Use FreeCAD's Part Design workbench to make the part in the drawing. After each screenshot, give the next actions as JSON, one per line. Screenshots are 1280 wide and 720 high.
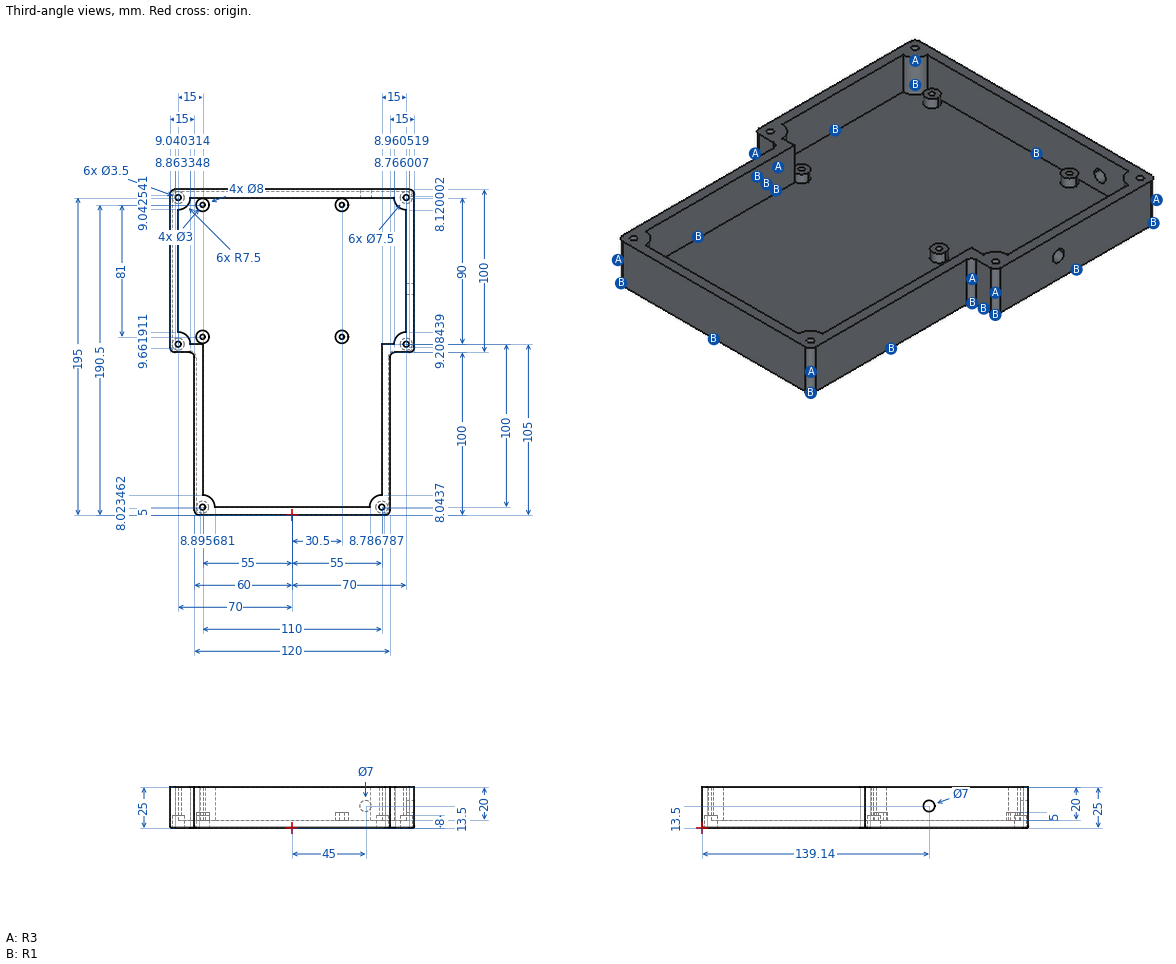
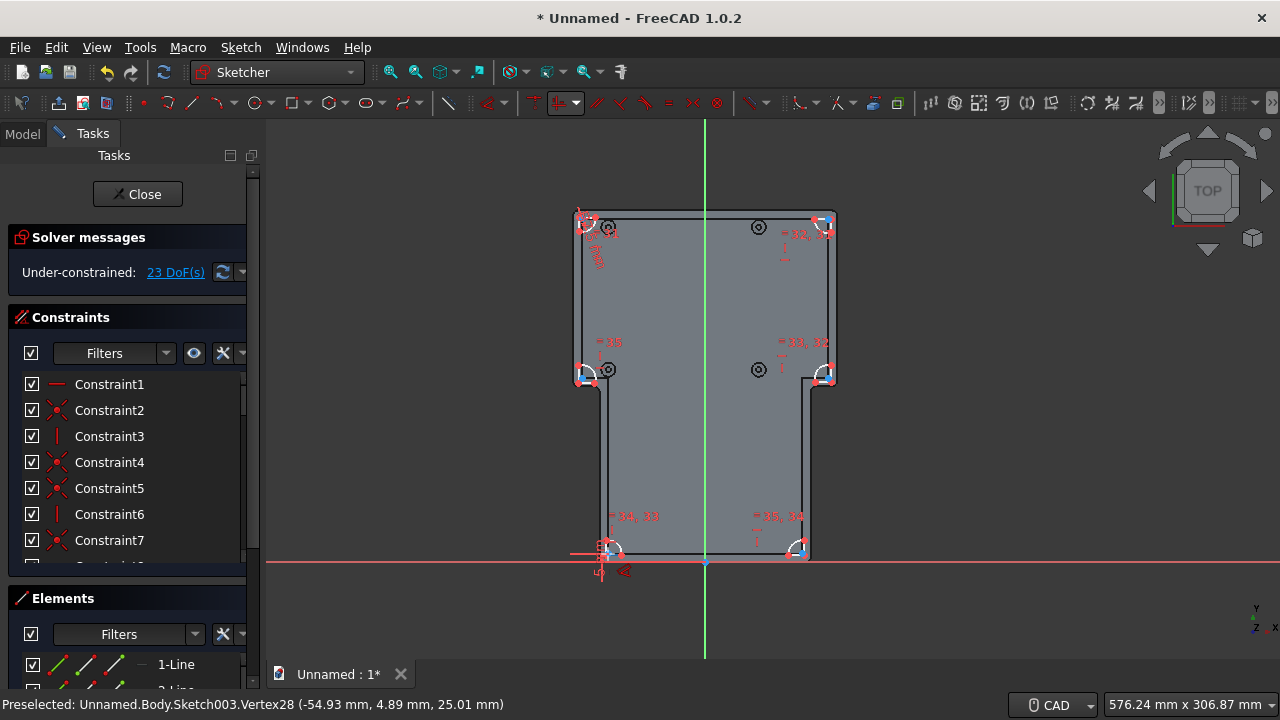
{"action": "scroll", "coordinate": [802, 554], "scroll_direction": "up", "scroll_amount": 8}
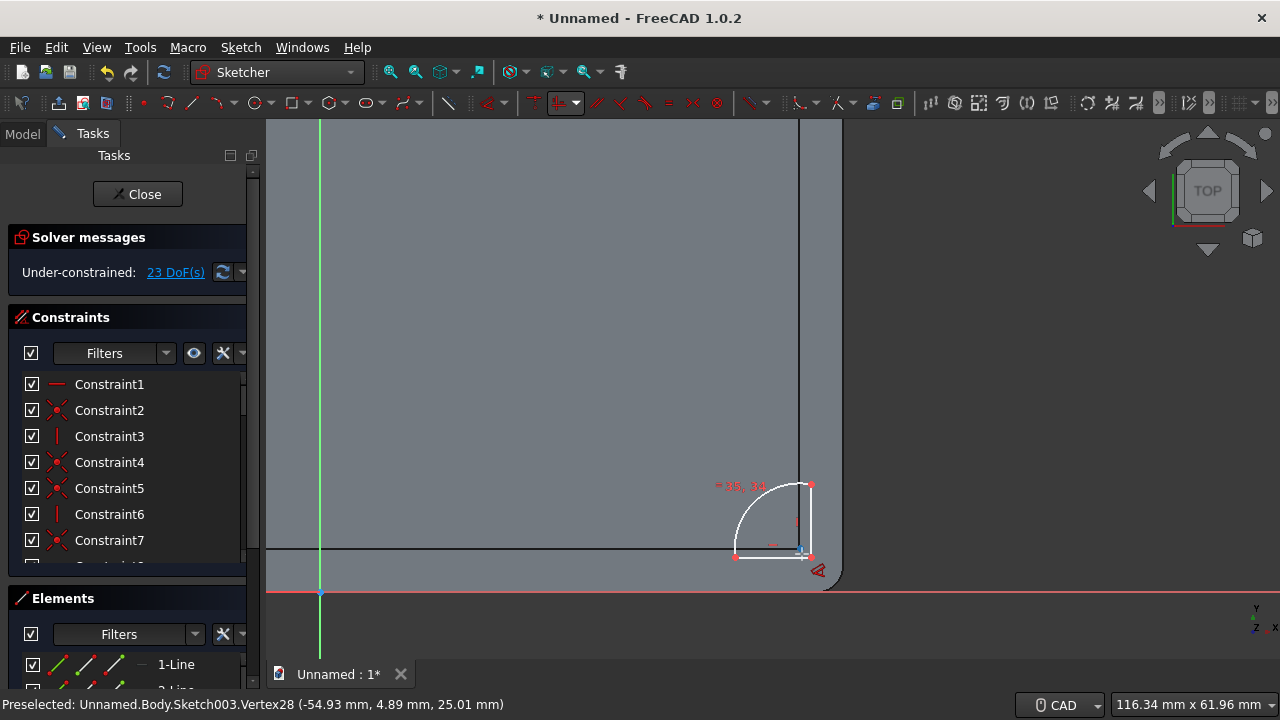
{"action": "left_click", "coordinate": [800, 549]}
{"action": "left_click", "coordinate": [834, 571]}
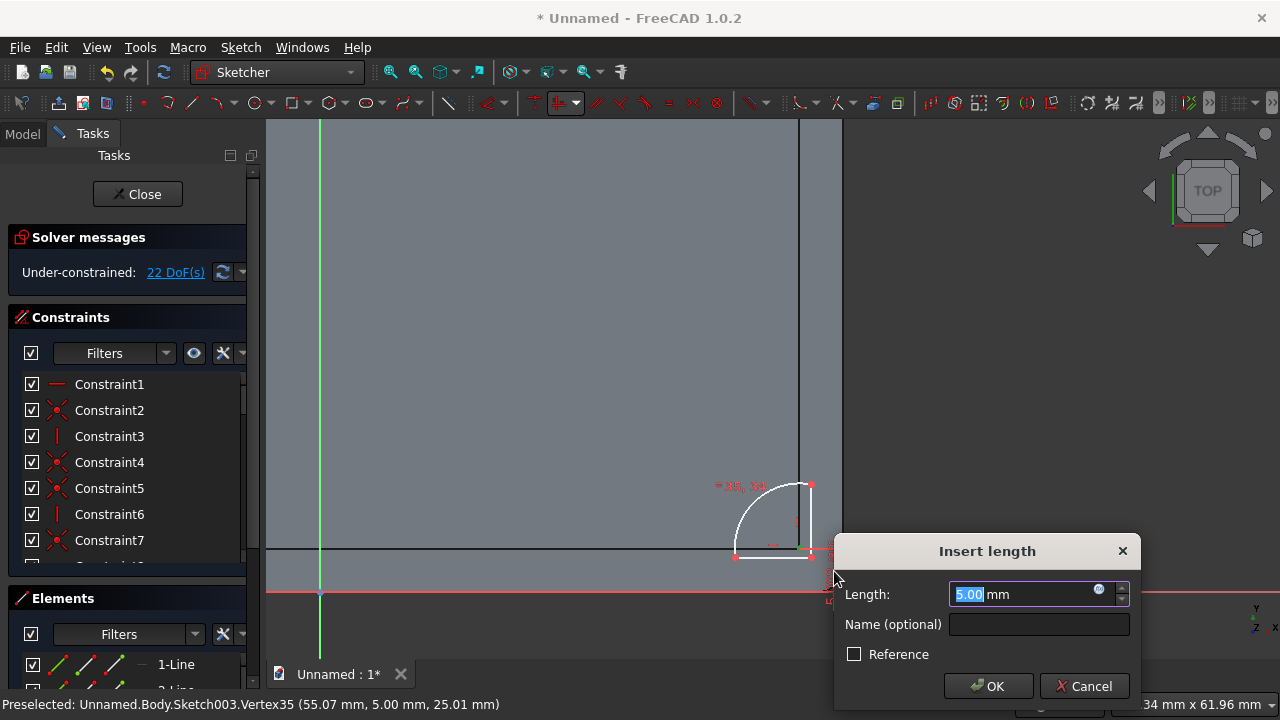
{"action": "type", "text": "5"}
{"action": "key", "text": "Return"}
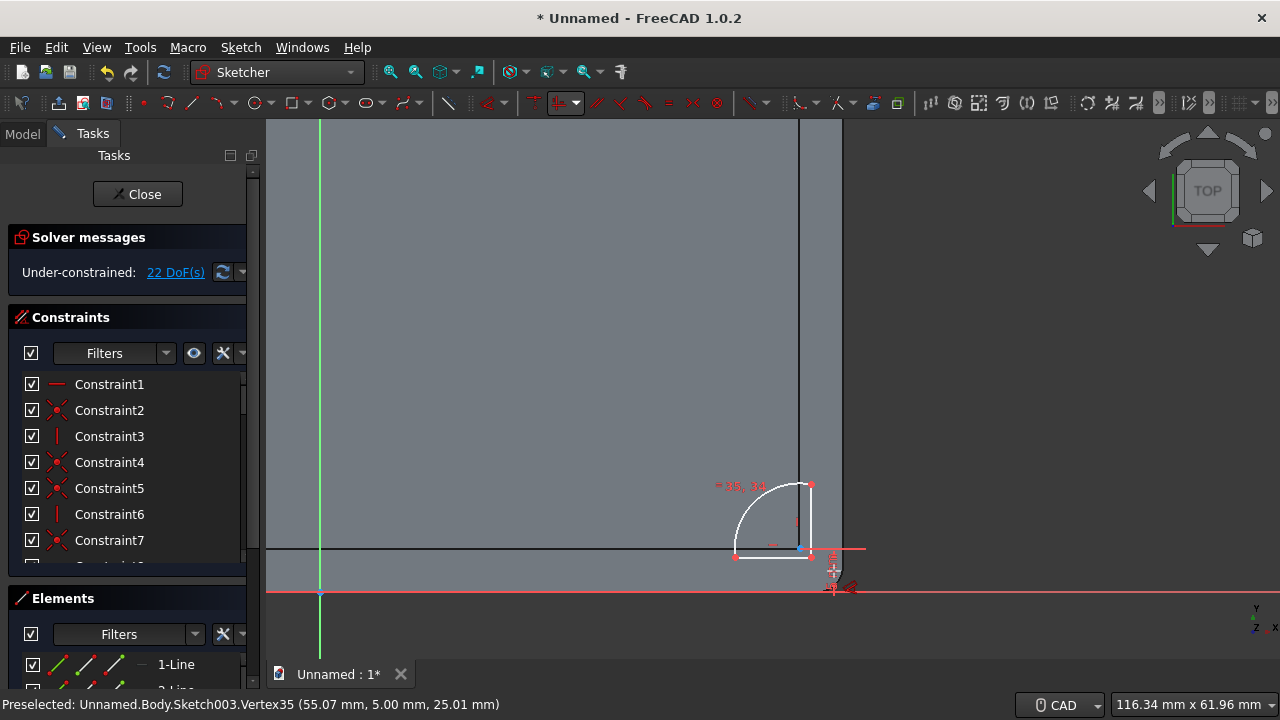
{"action": "scroll", "coordinate": [802, 554], "scroll_direction": "down", "scroll_amount": 8}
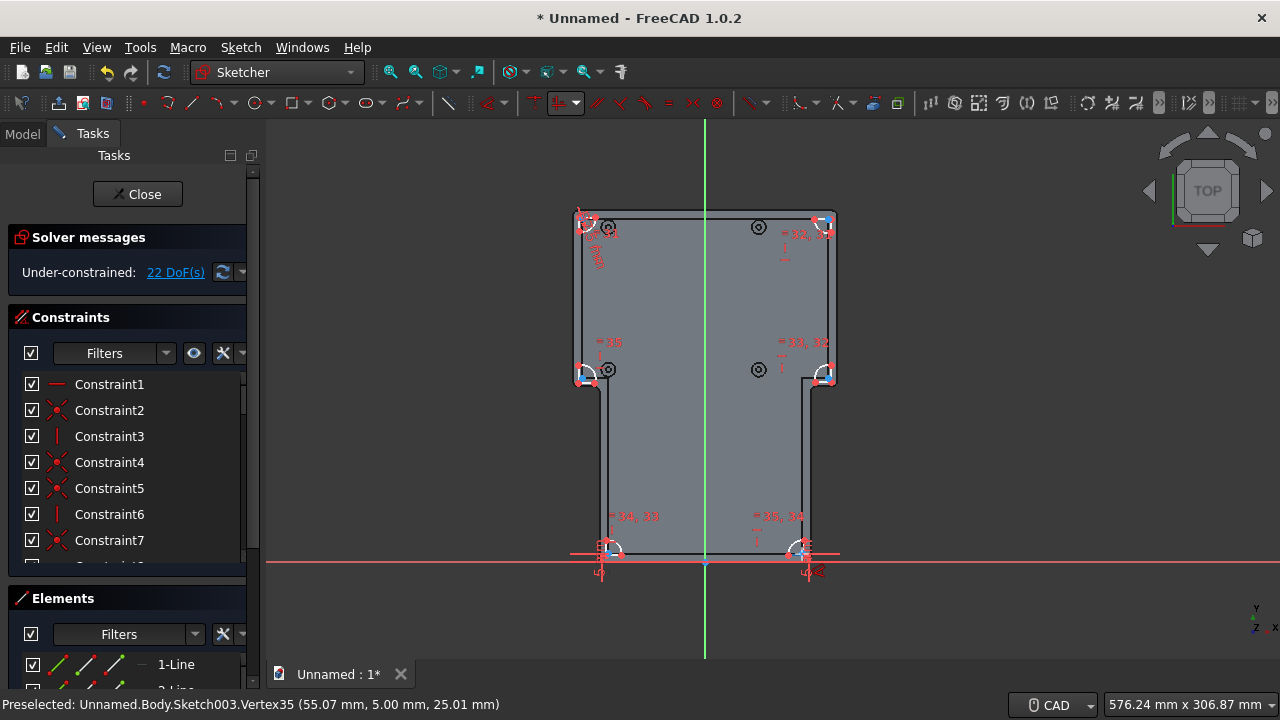
{"action": "scroll", "coordinate": [582, 219], "scroll_direction": "up", "scroll_amount": 7}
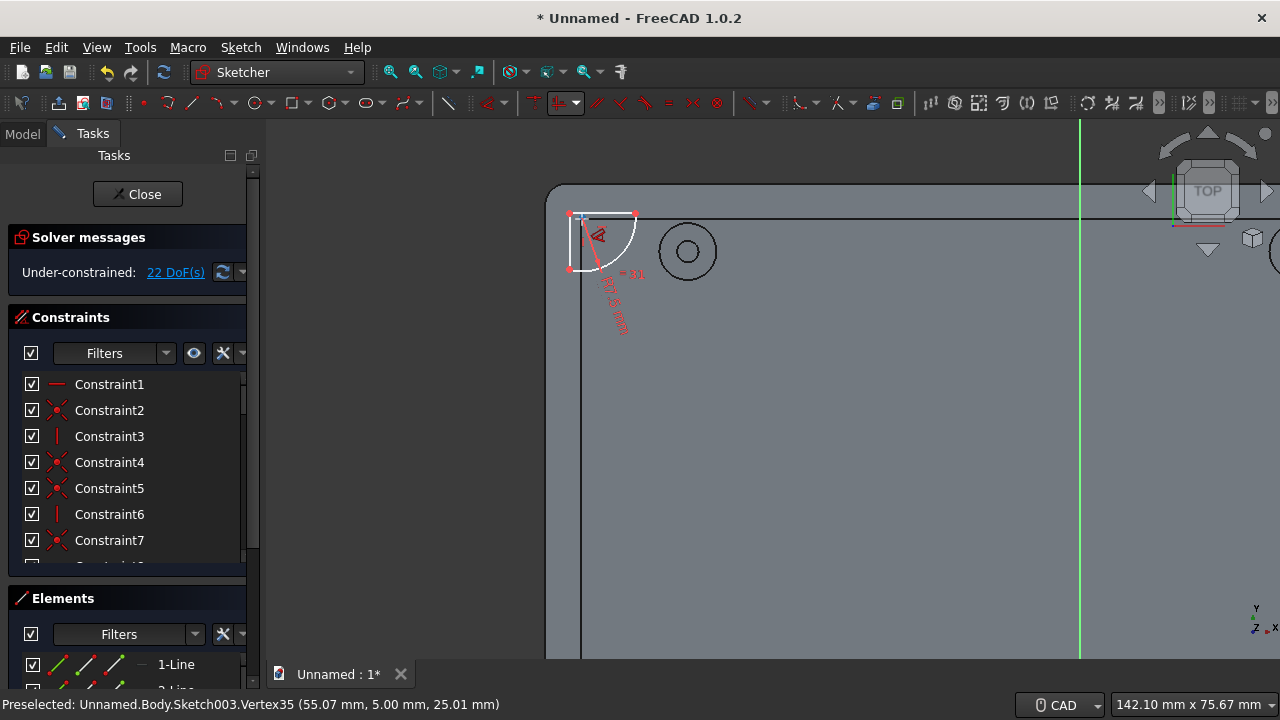
{"action": "left_click", "coordinate": [582, 218]}
{"action": "left_click", "coordinate": [831, 184]}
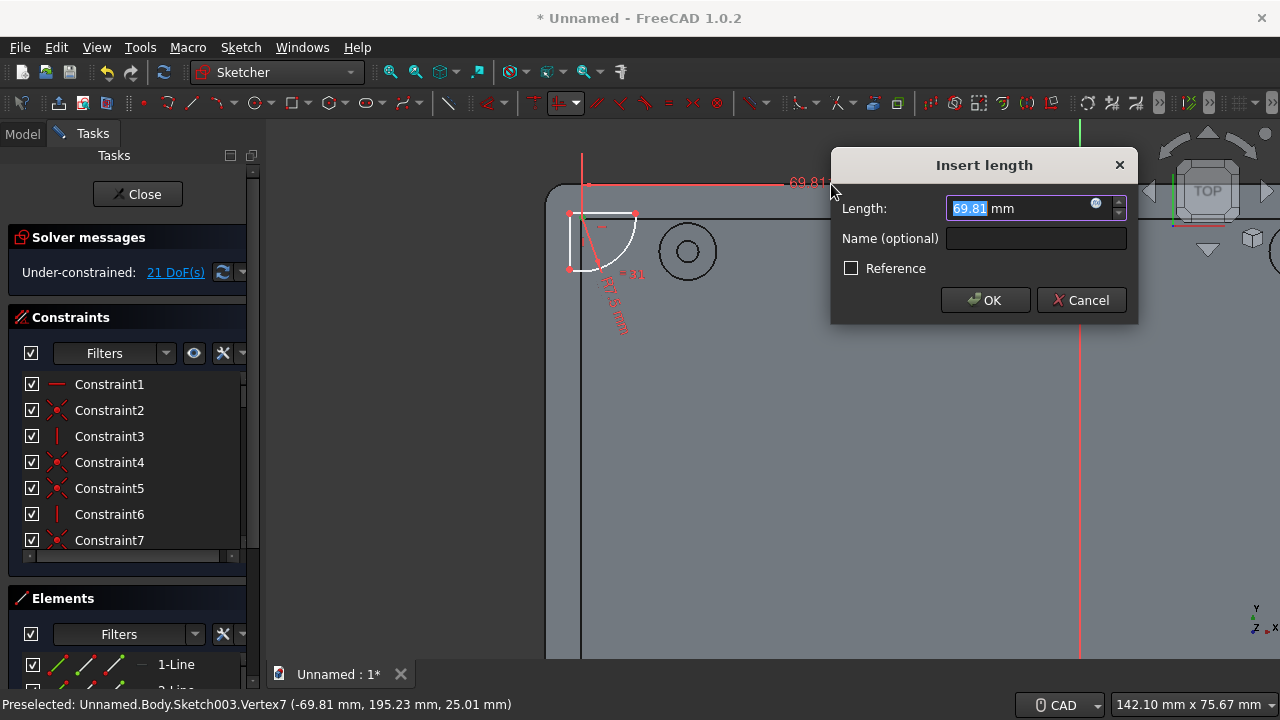
{"action": "type", "text": "70"}
{"action": "key", "text": "Return"}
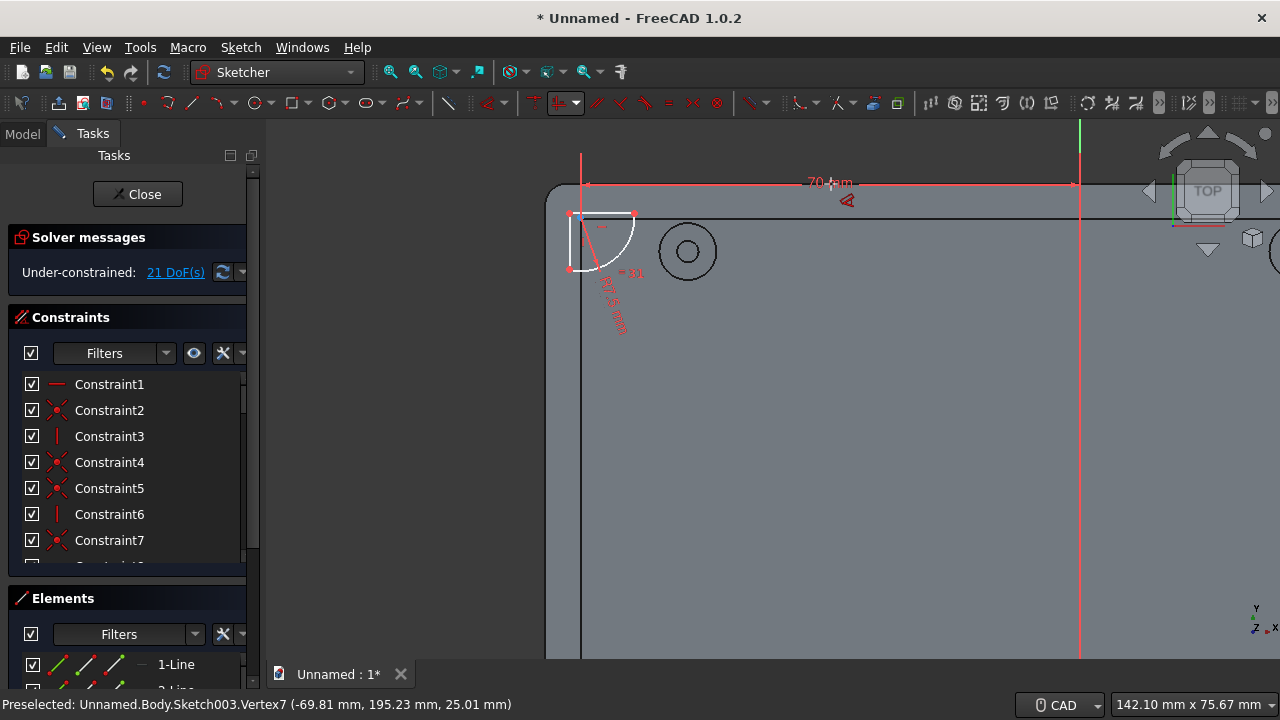
{"action": "scroll", "coordinate": [582, 219], "scroll_direction": "down", "scroll_amount": 7}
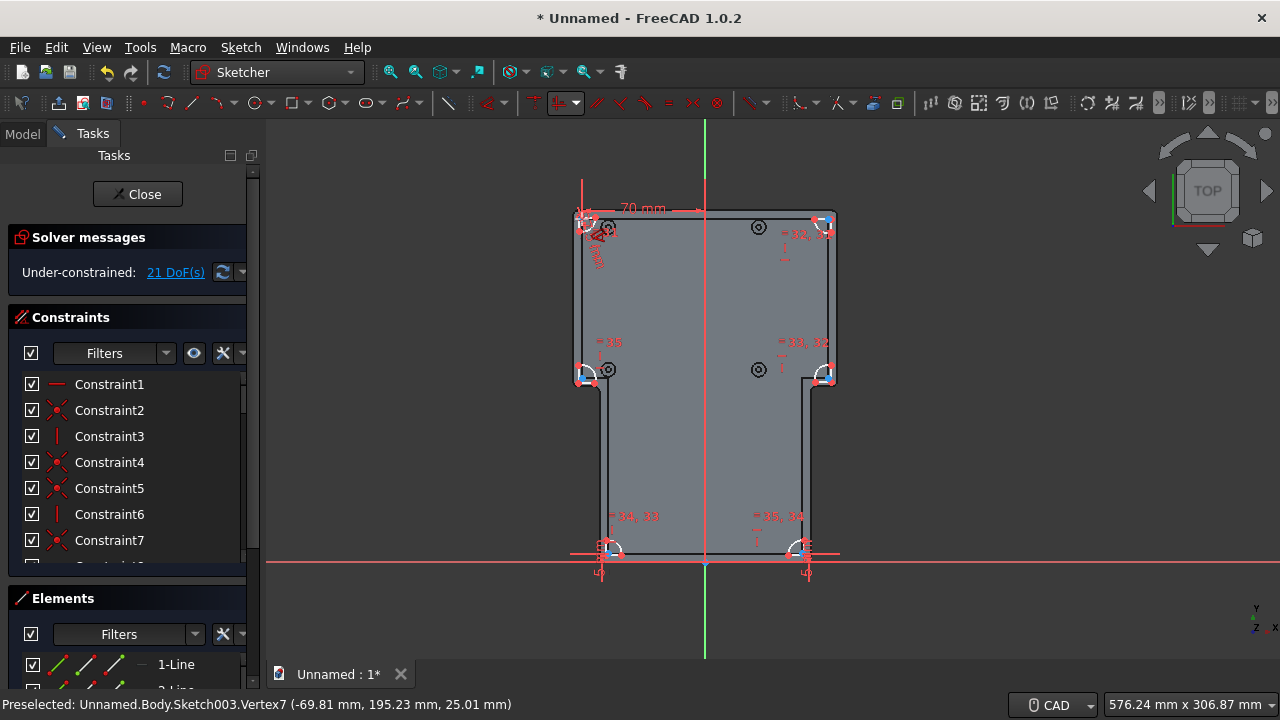
{"action": "scroll", "coordinate": [828, 220], "scroll_direction": "up", "scroll_amount": 7}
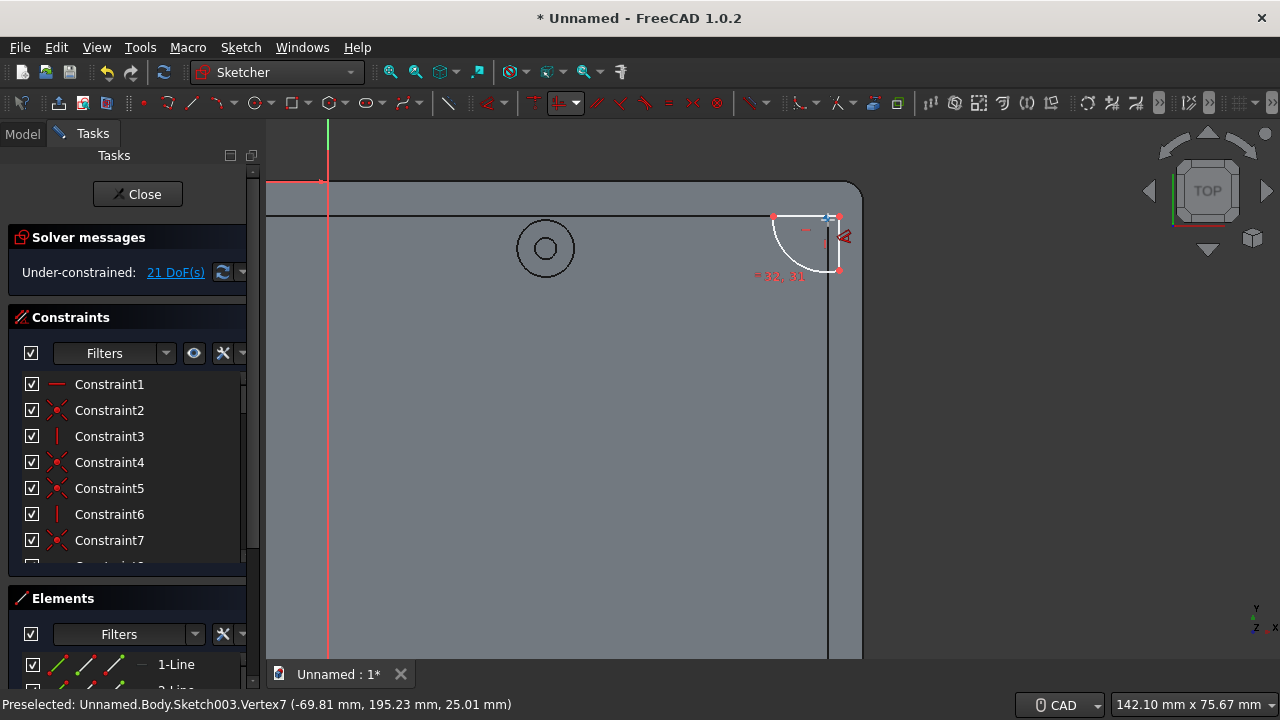
{"action": "left_click", "coordinate": [827, 219]}
{"action": "left_click", "coordinate": [577, 185]}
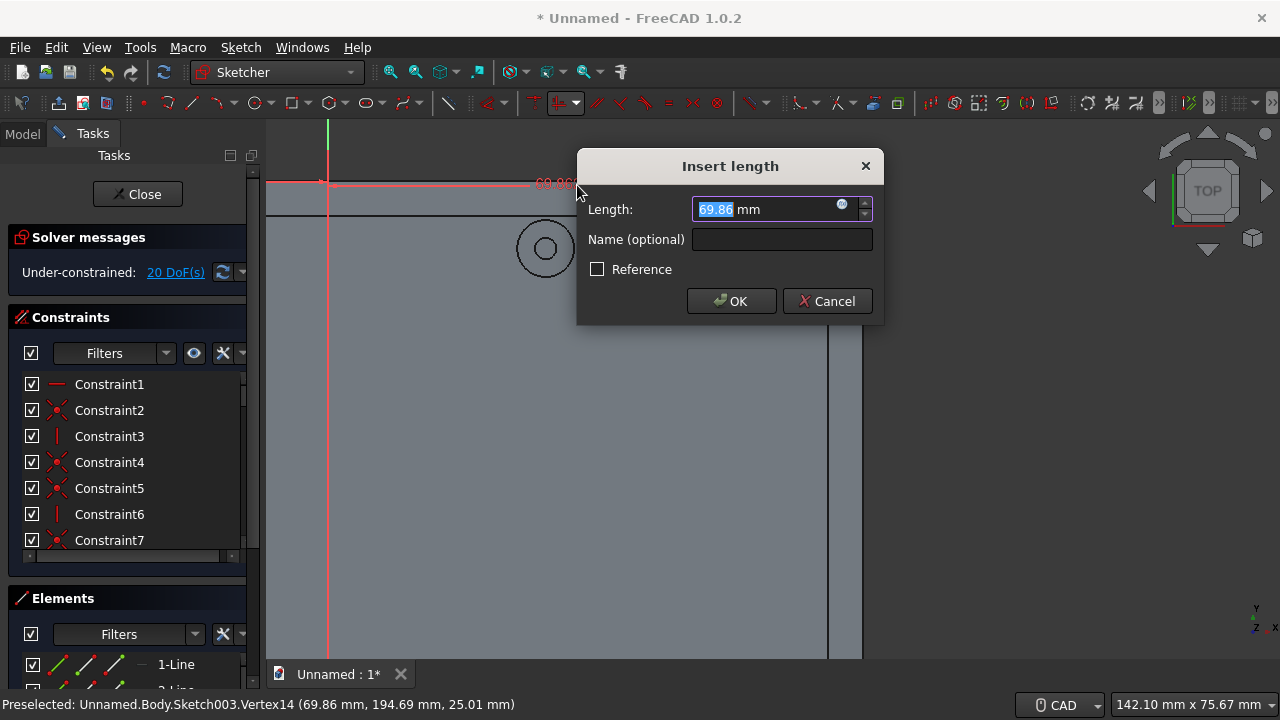
{"action": "type", "text": "70"}
{"action": "key", "text": "Return"}